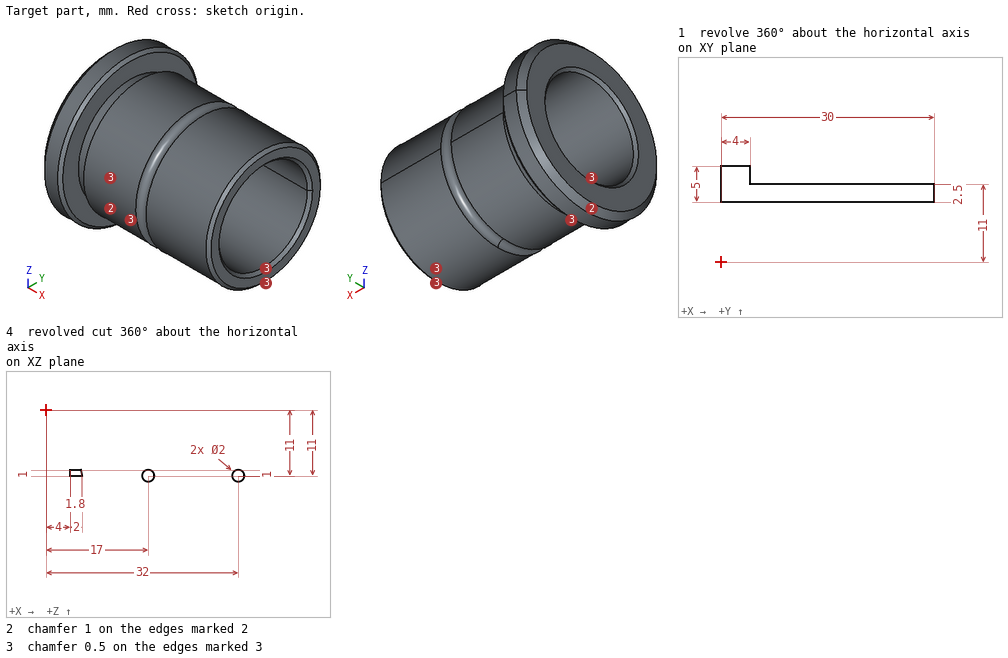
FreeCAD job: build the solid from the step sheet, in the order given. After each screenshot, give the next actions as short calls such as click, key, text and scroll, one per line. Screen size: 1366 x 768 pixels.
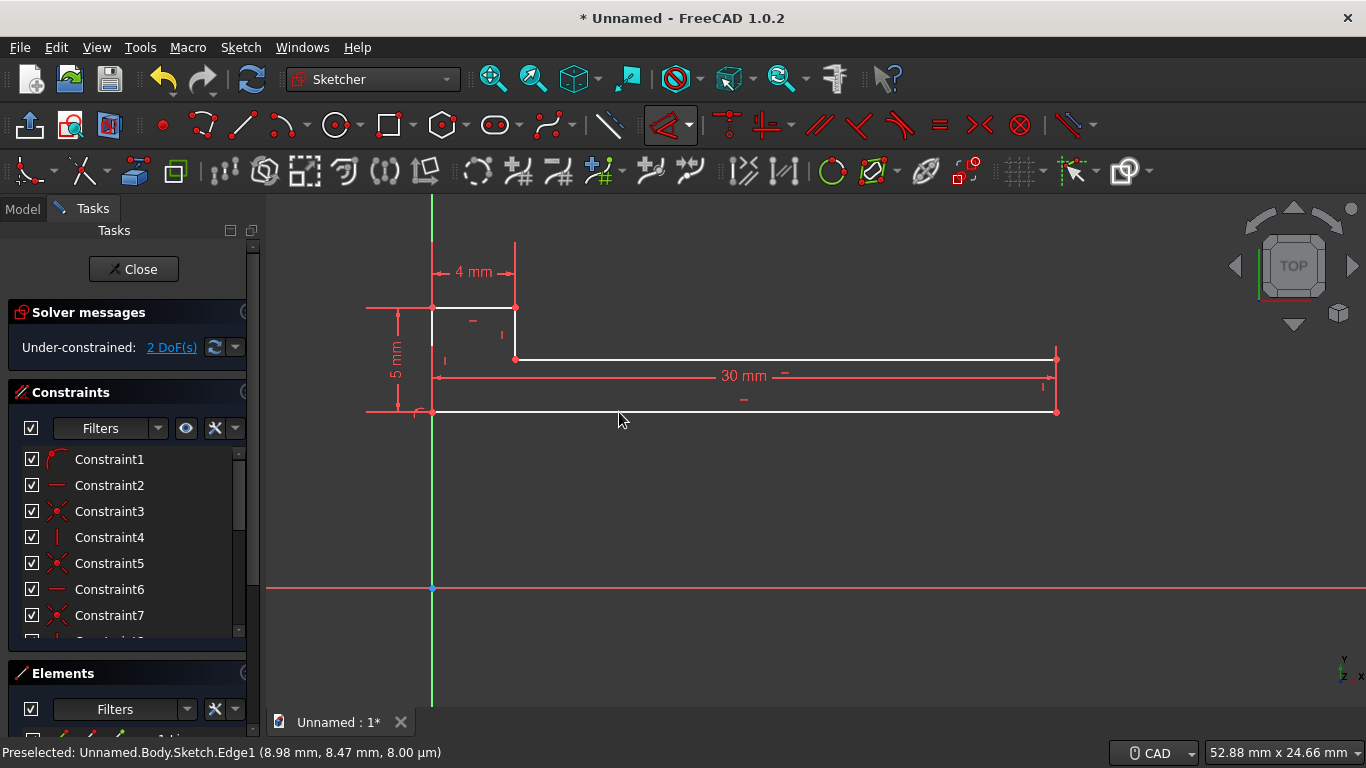
click(1056, 396)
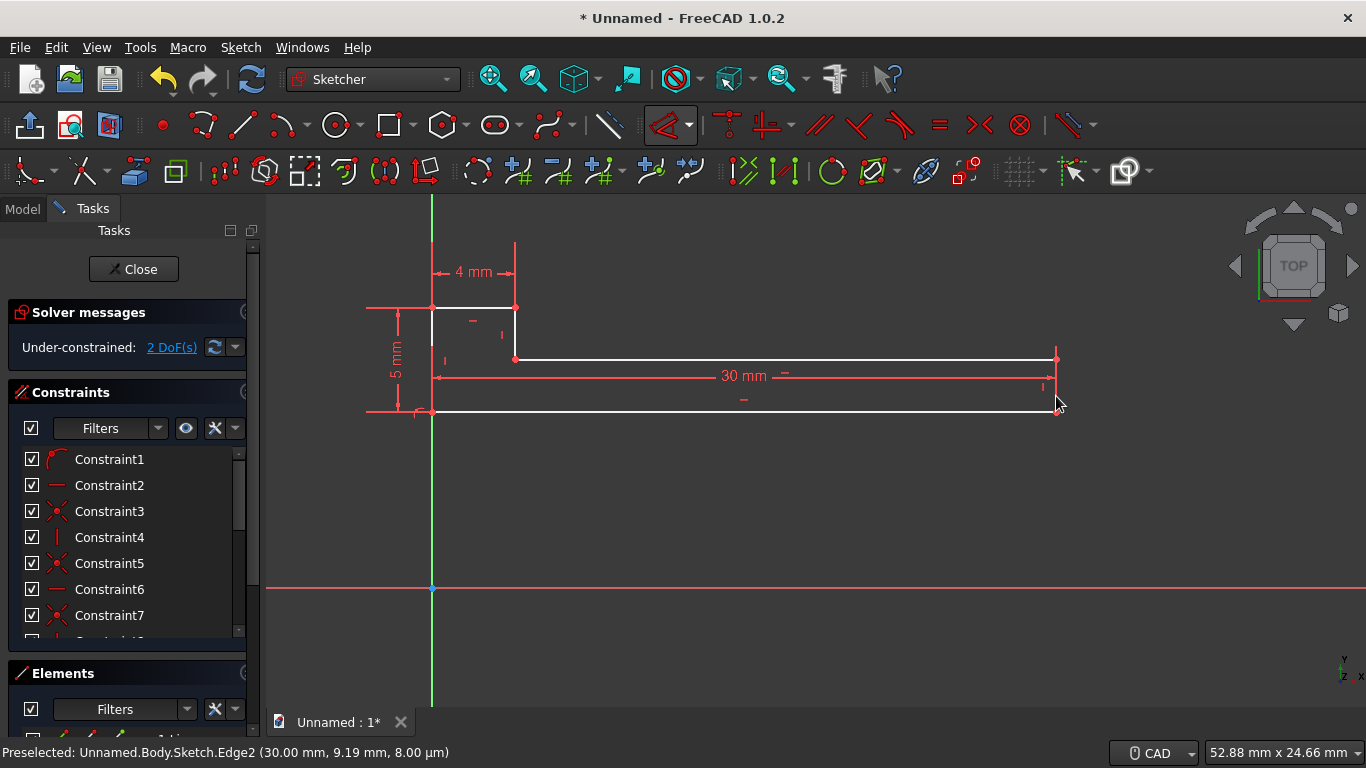
key(i)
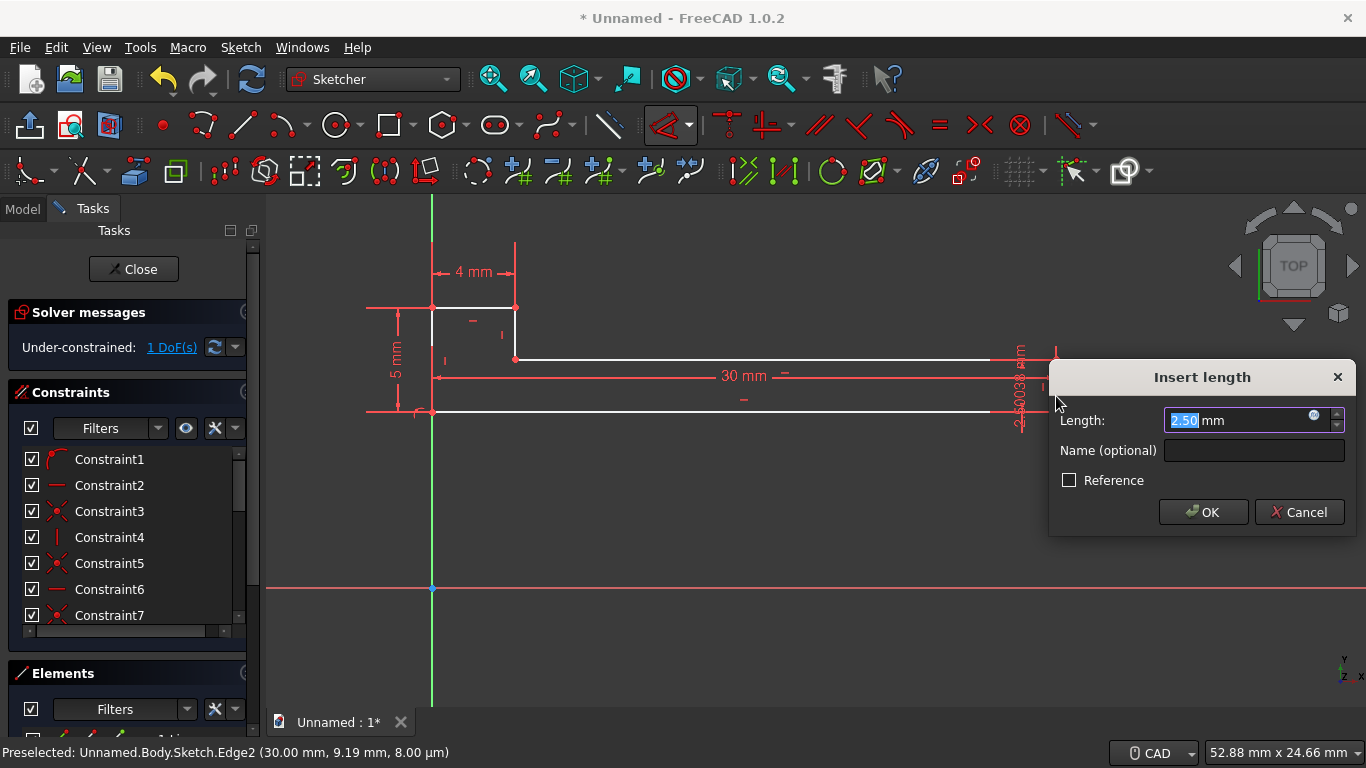
text(2.5)
key(Return)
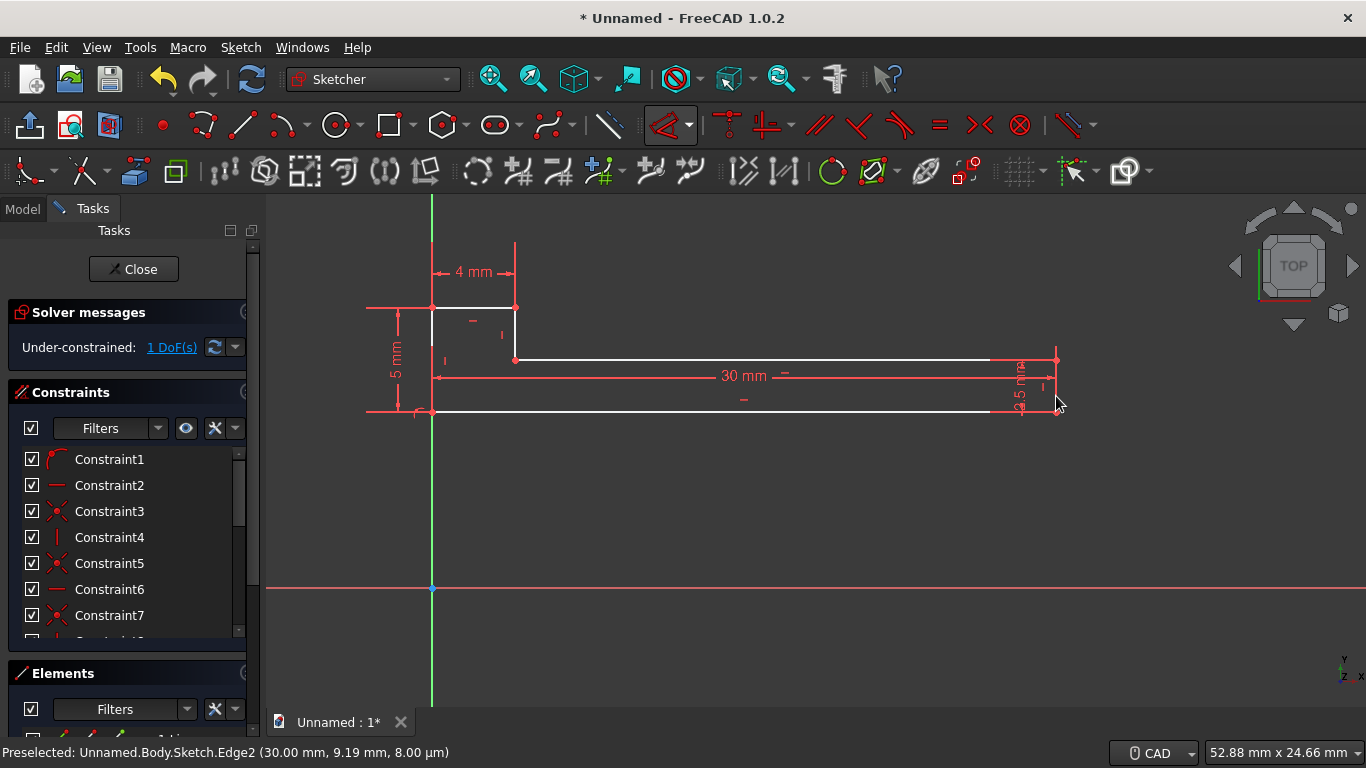
click(1056, 360)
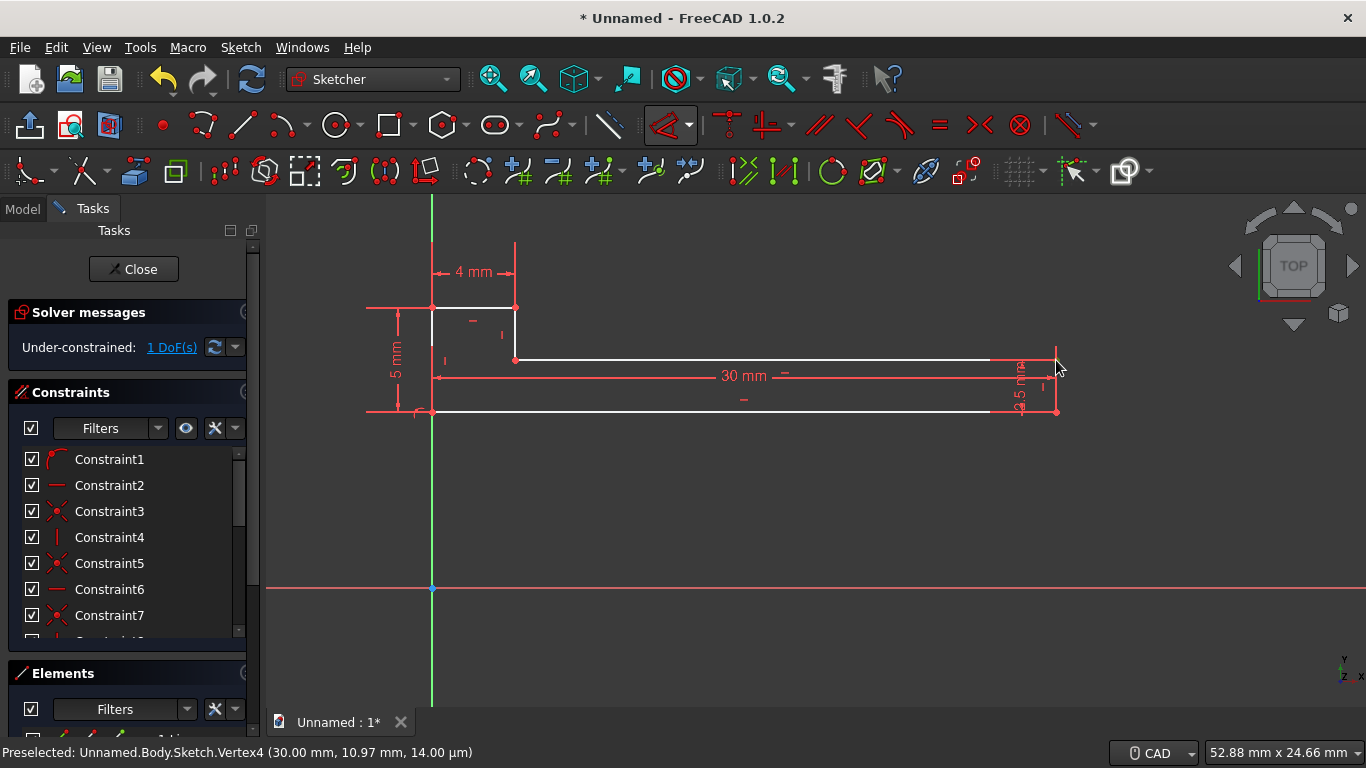
key(i)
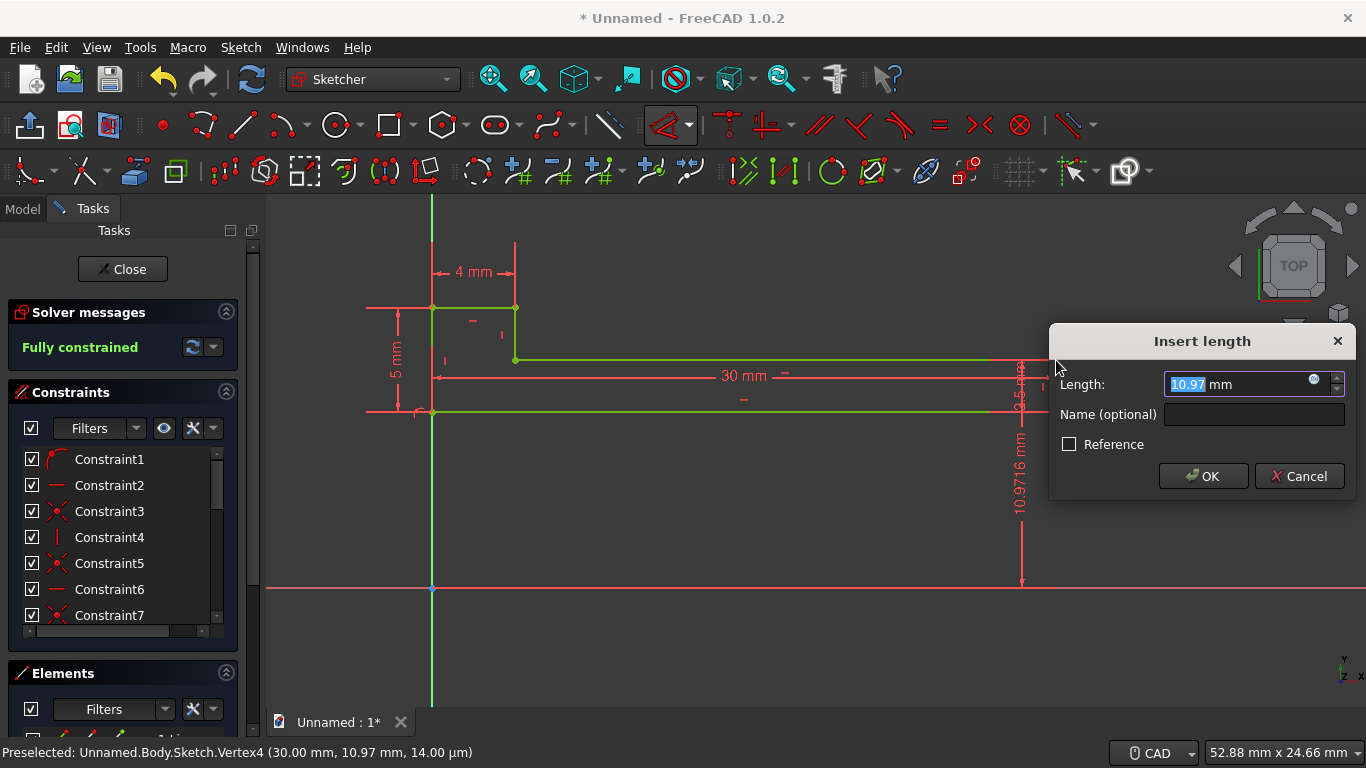
text(11)
key(Return)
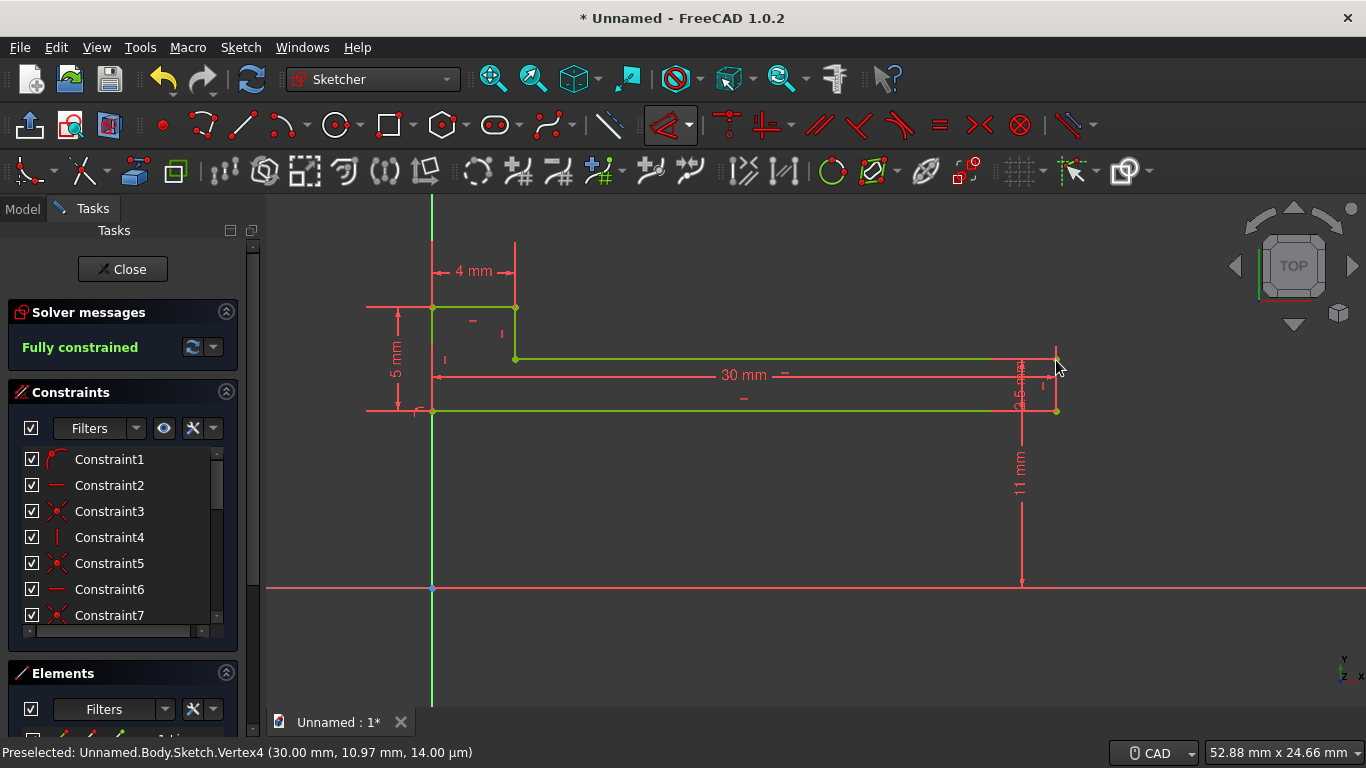
click(123, 269)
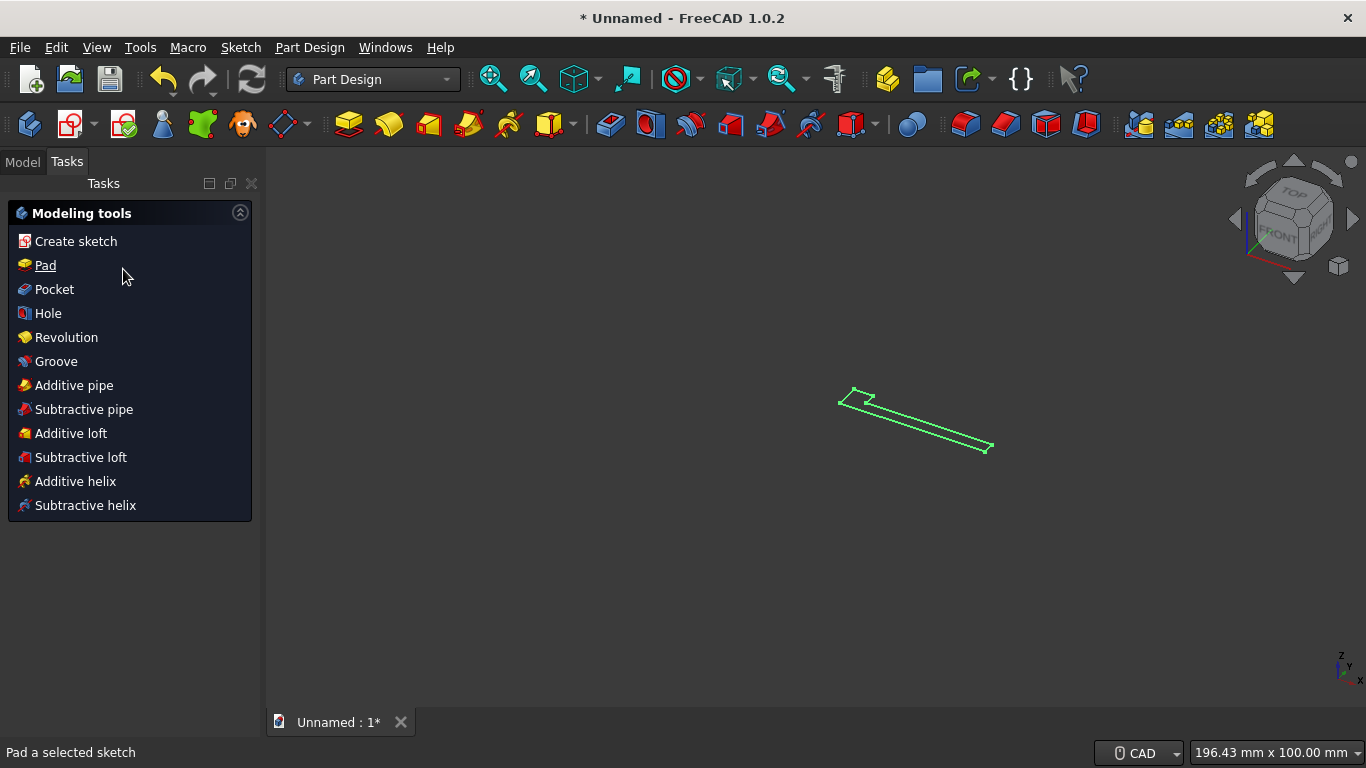
click(390, 124)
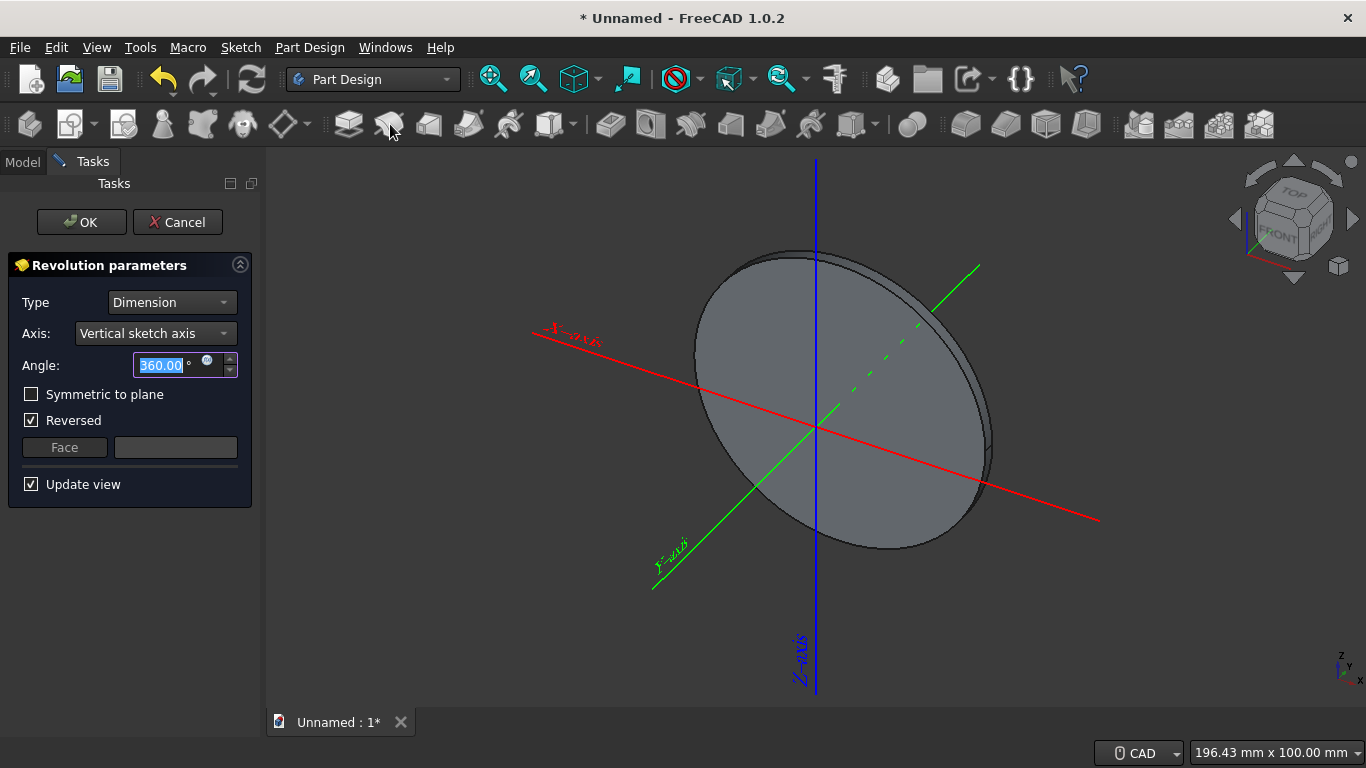
click(156, 334)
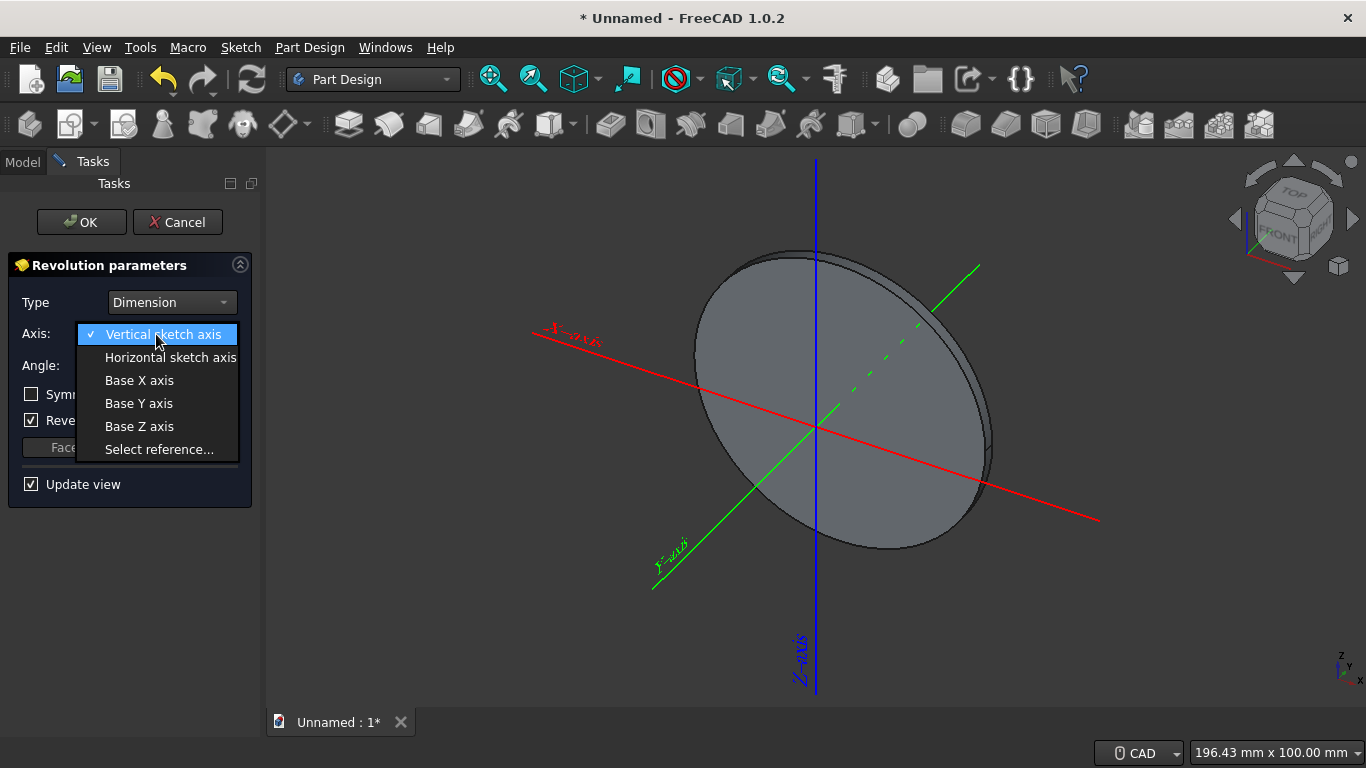
click(156, 358)